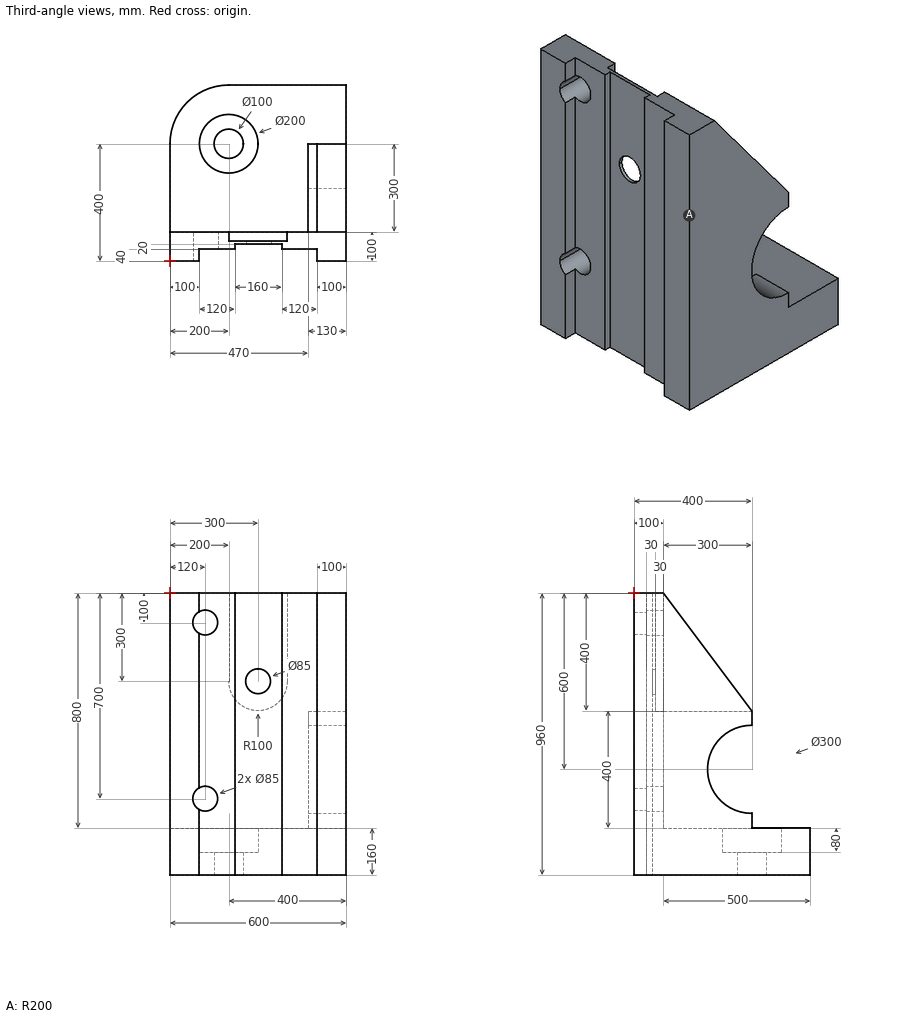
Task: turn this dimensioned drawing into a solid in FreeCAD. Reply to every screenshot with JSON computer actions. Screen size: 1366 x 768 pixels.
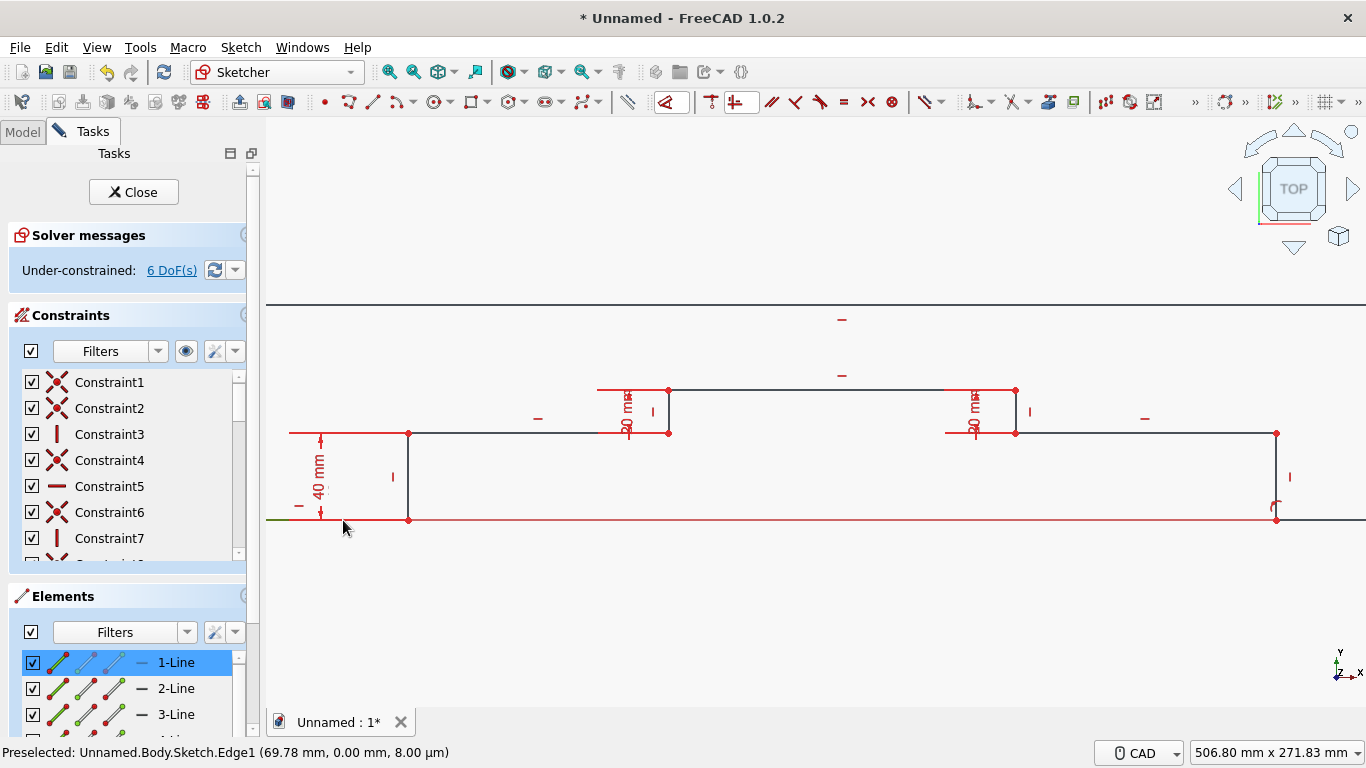
{"action": "left_click", "coordinate": [684, 102]}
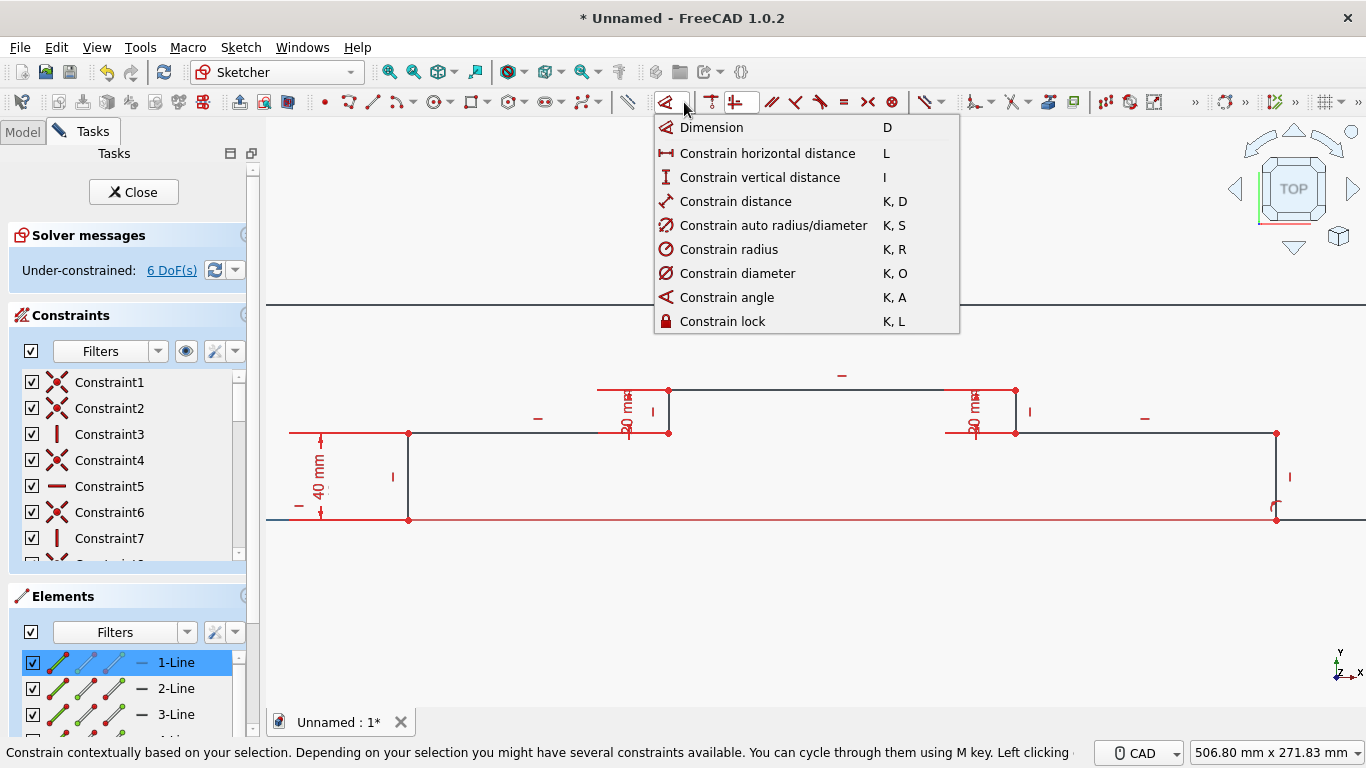
{"action": "left_click", "coordinate": [807, 153]}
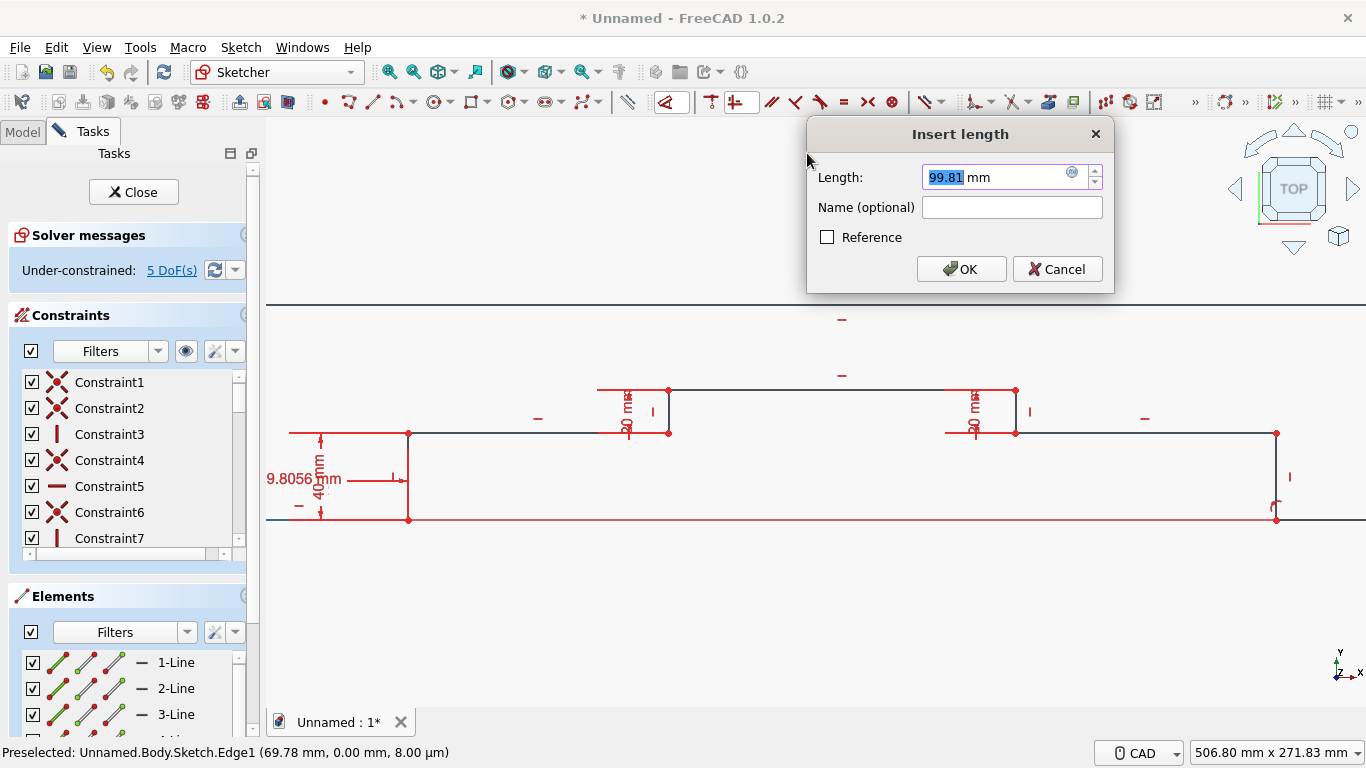
{"action": "type", "text": "100"}
{"action": "key", "text": "Return"}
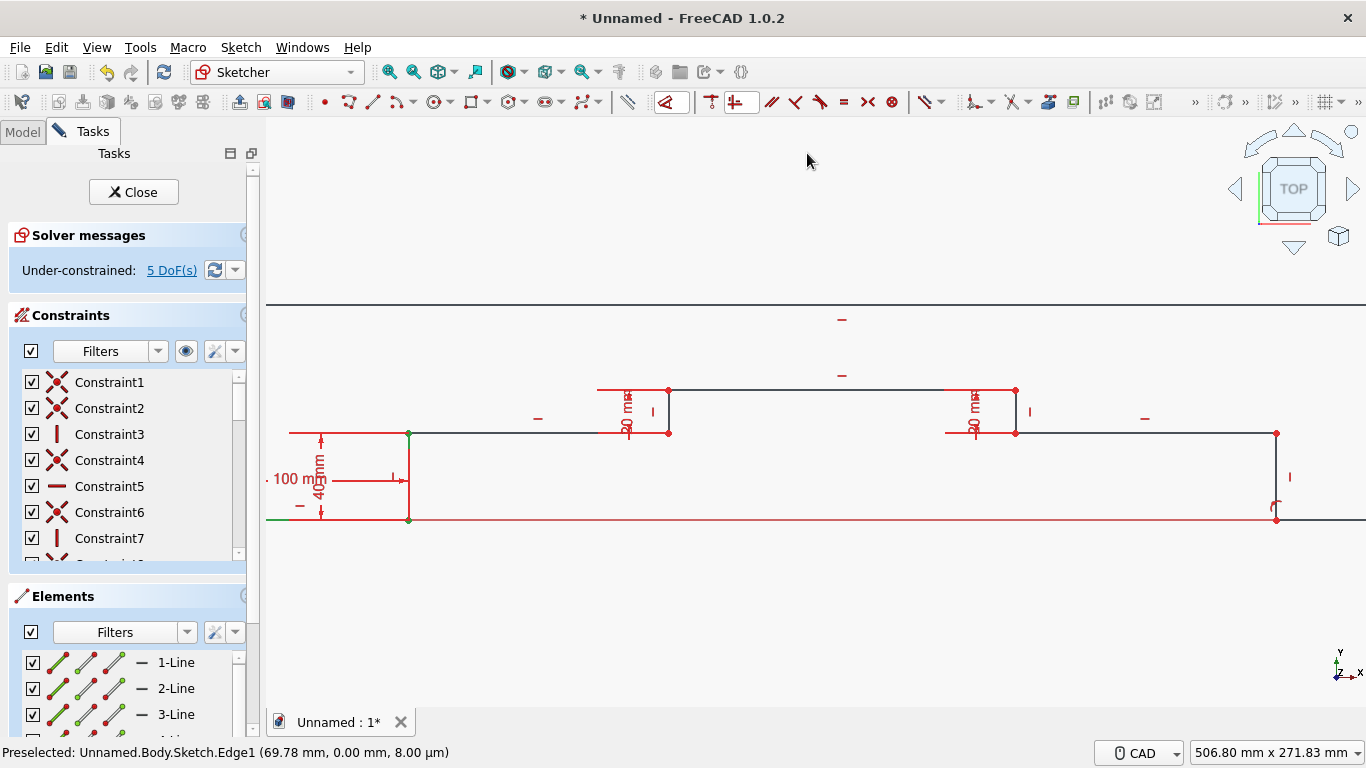
{"action": "left_click", "coordinate": [487, 433]}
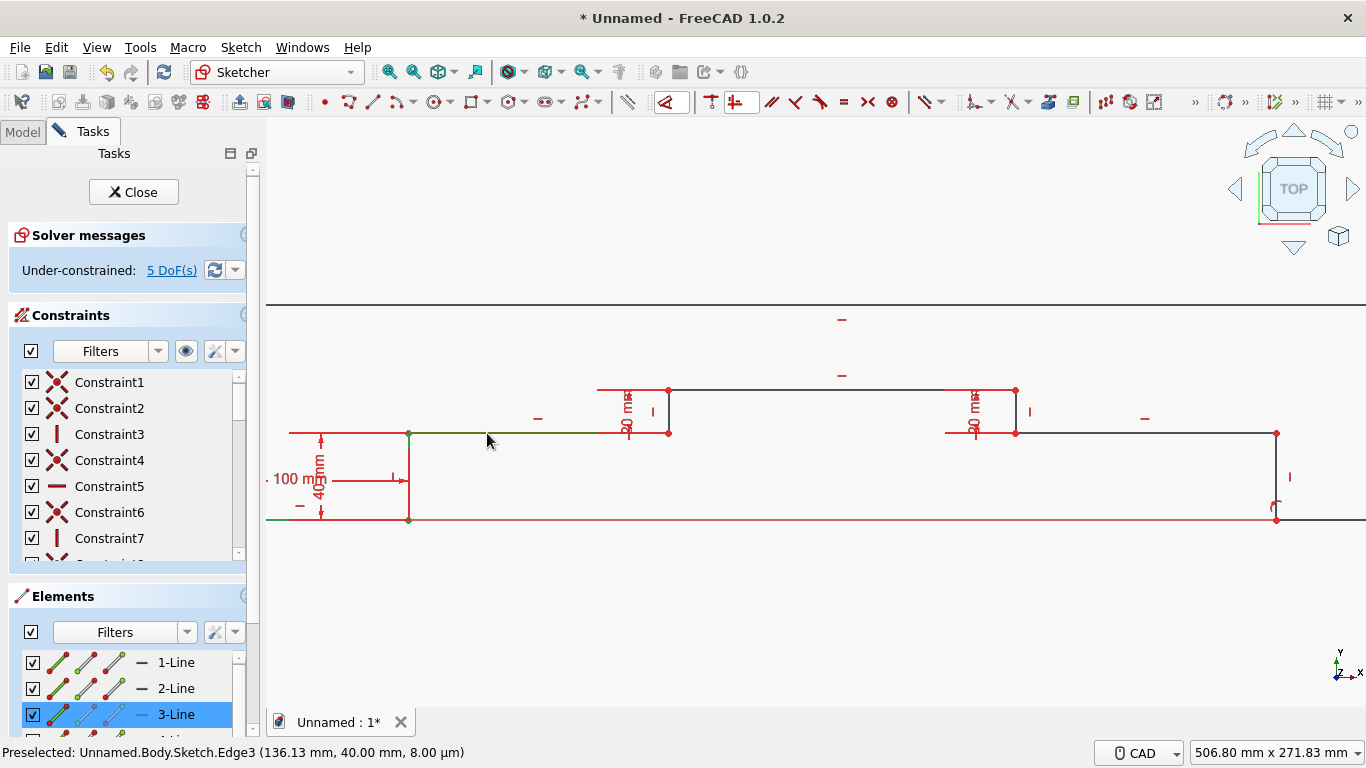
{"action": "left_click", "coordinate": [684, 102]}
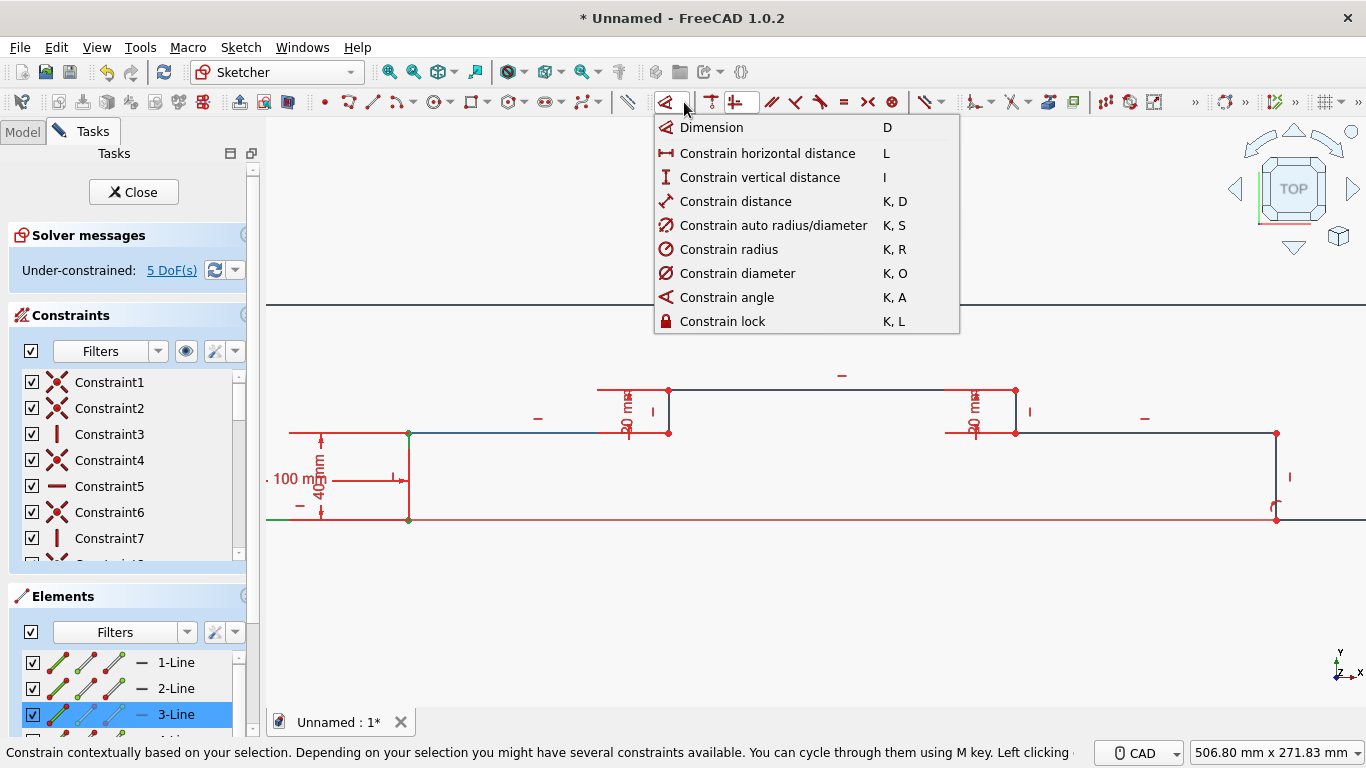
{"action": "left_click", "coordinate": [807, 153]}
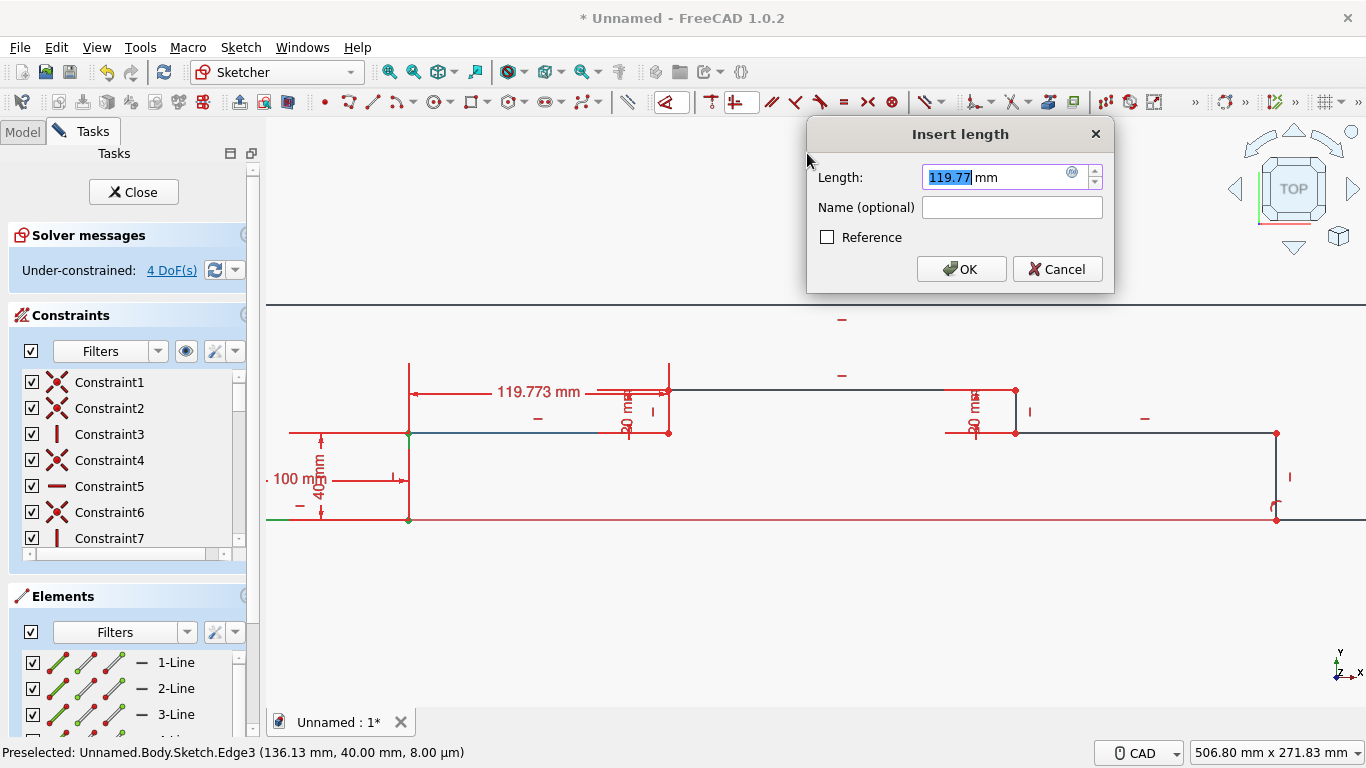
{"action": "type", "text": "120"}
{"action": "key", "text": "Return"}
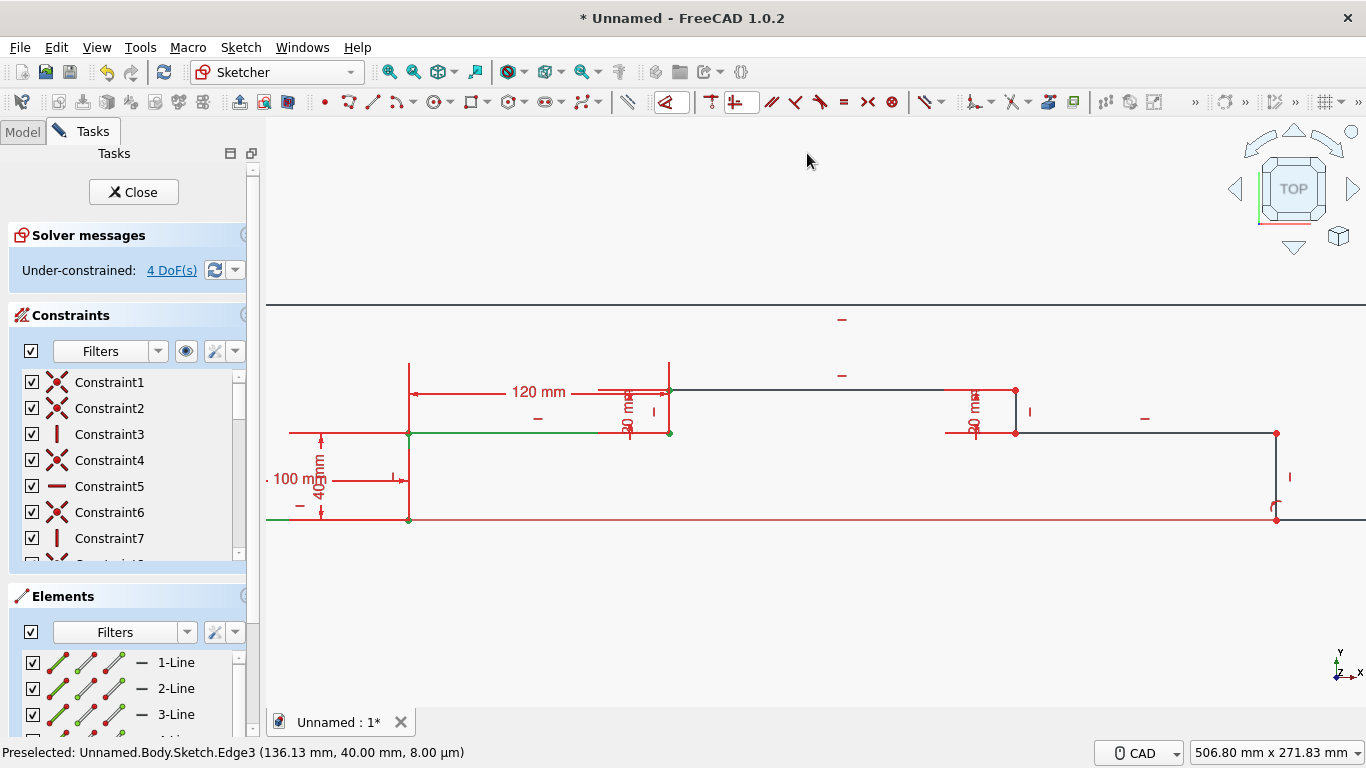
{"action": "left_click", "coordinate": [773, 390]}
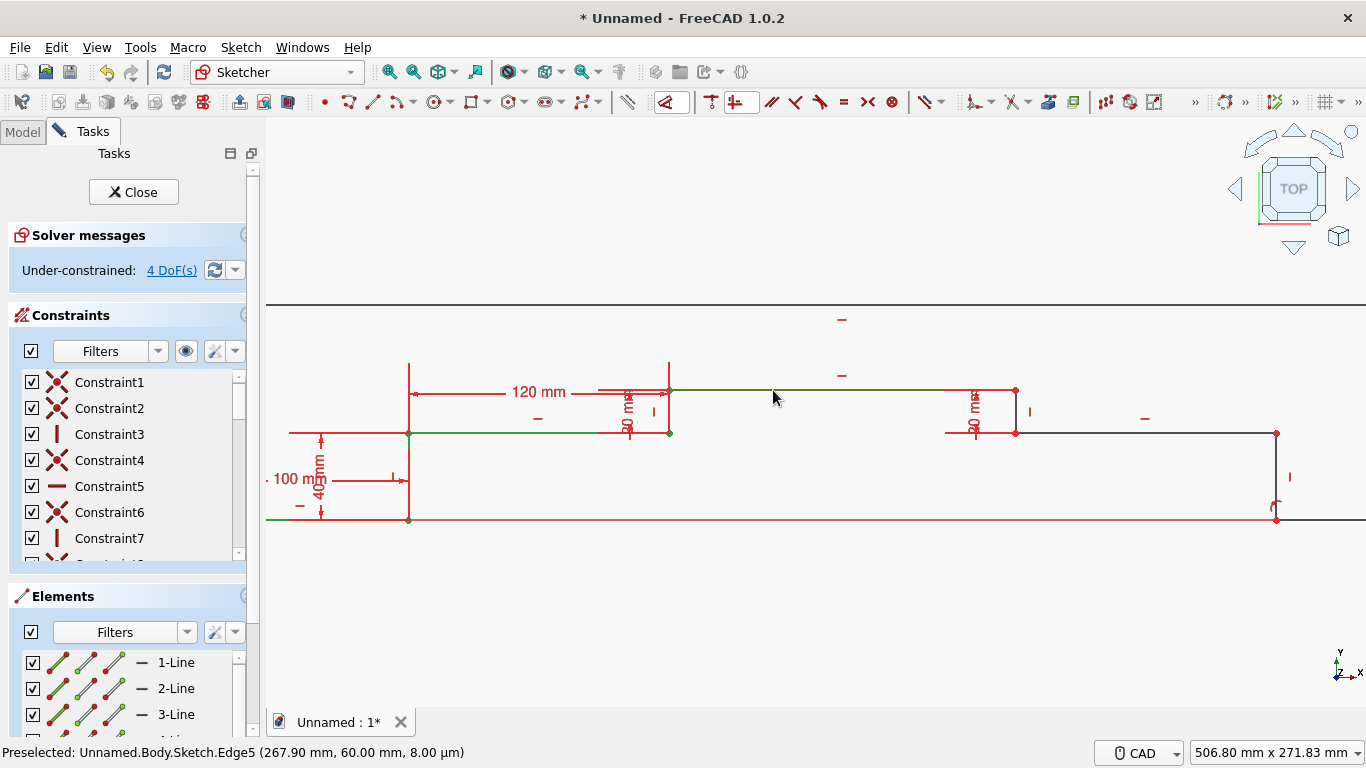
{"action": "key", "text": "l"}